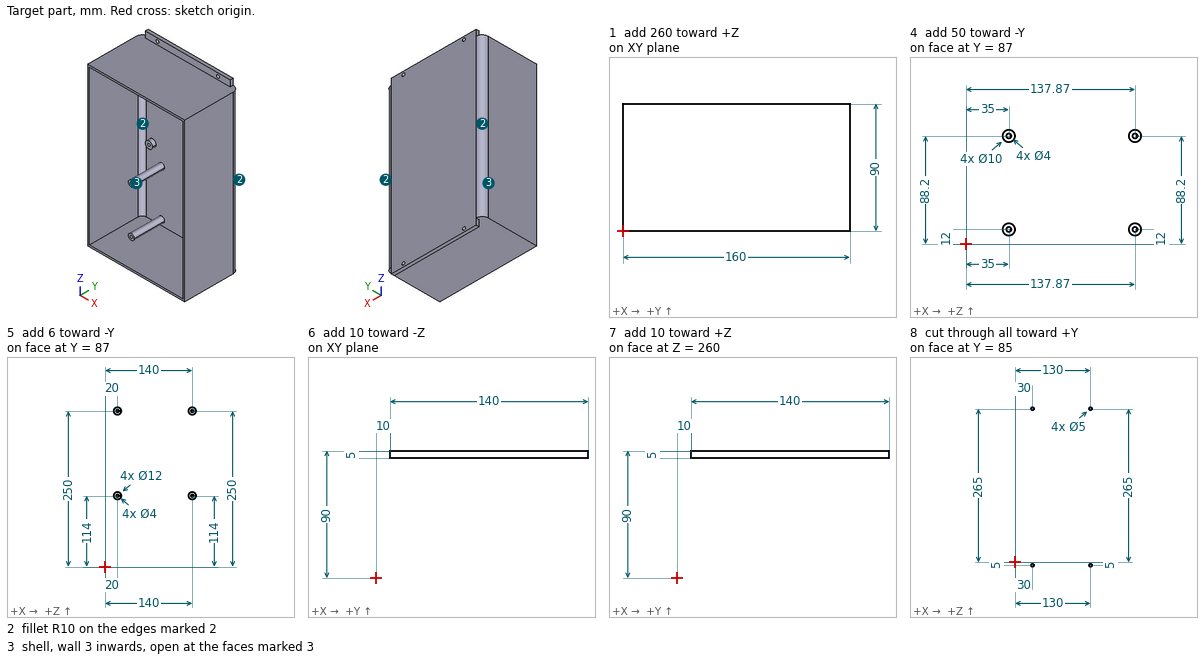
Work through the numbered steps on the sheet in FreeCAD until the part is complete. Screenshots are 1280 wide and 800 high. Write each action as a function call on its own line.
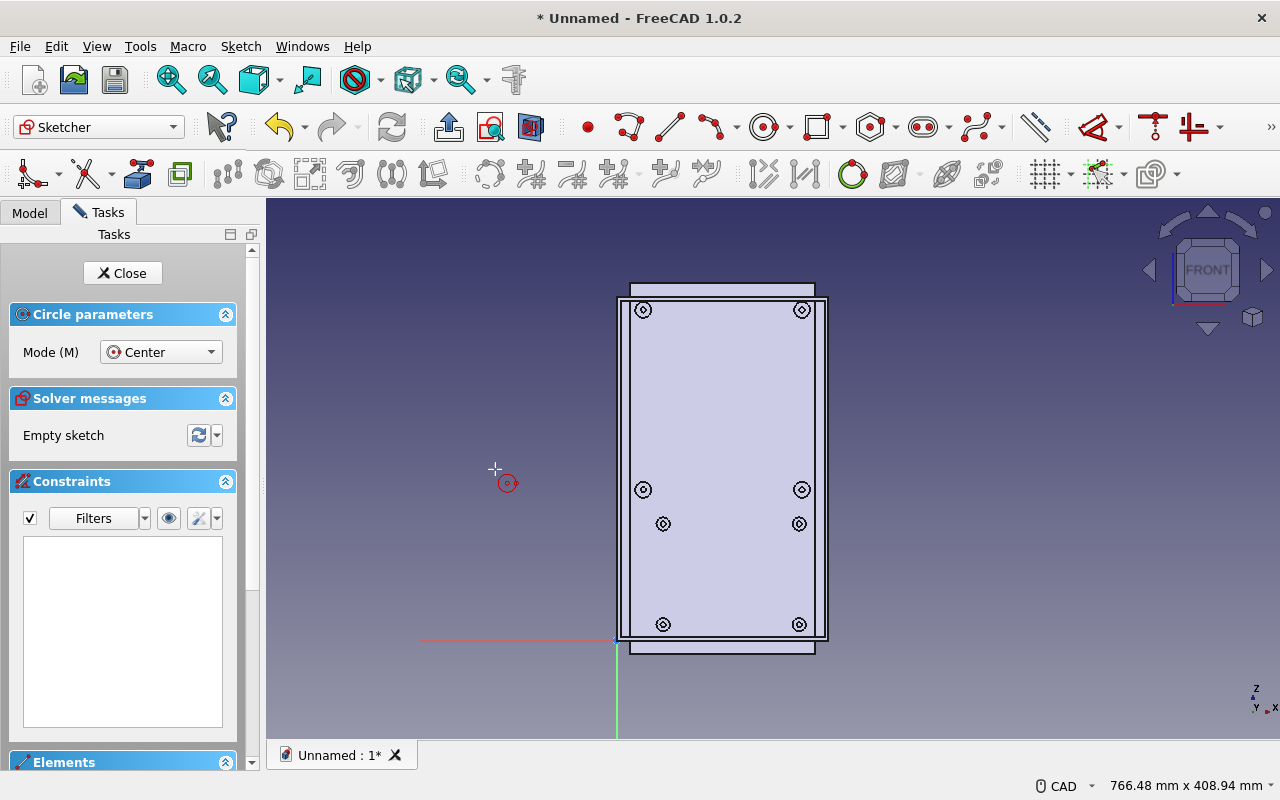
scroll(789, 290, up, 10)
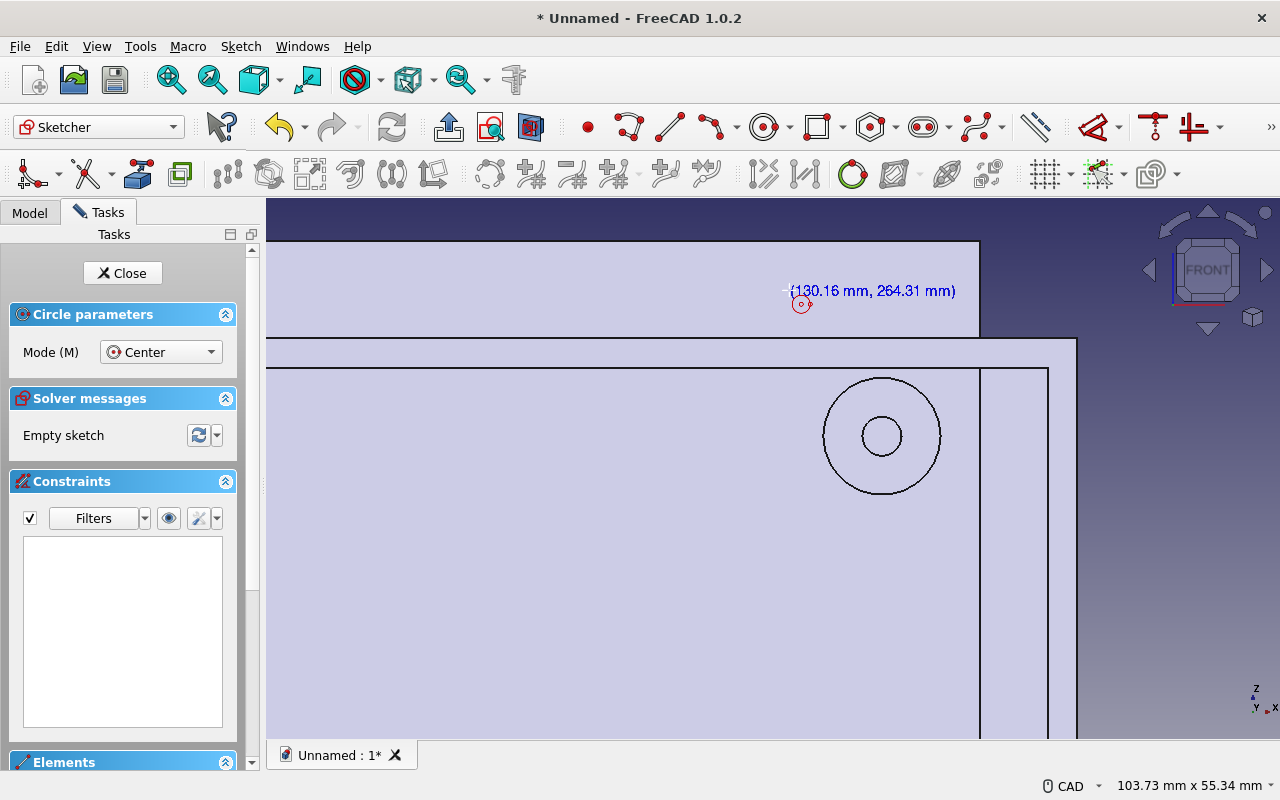
scroll(790, 290, down, 10)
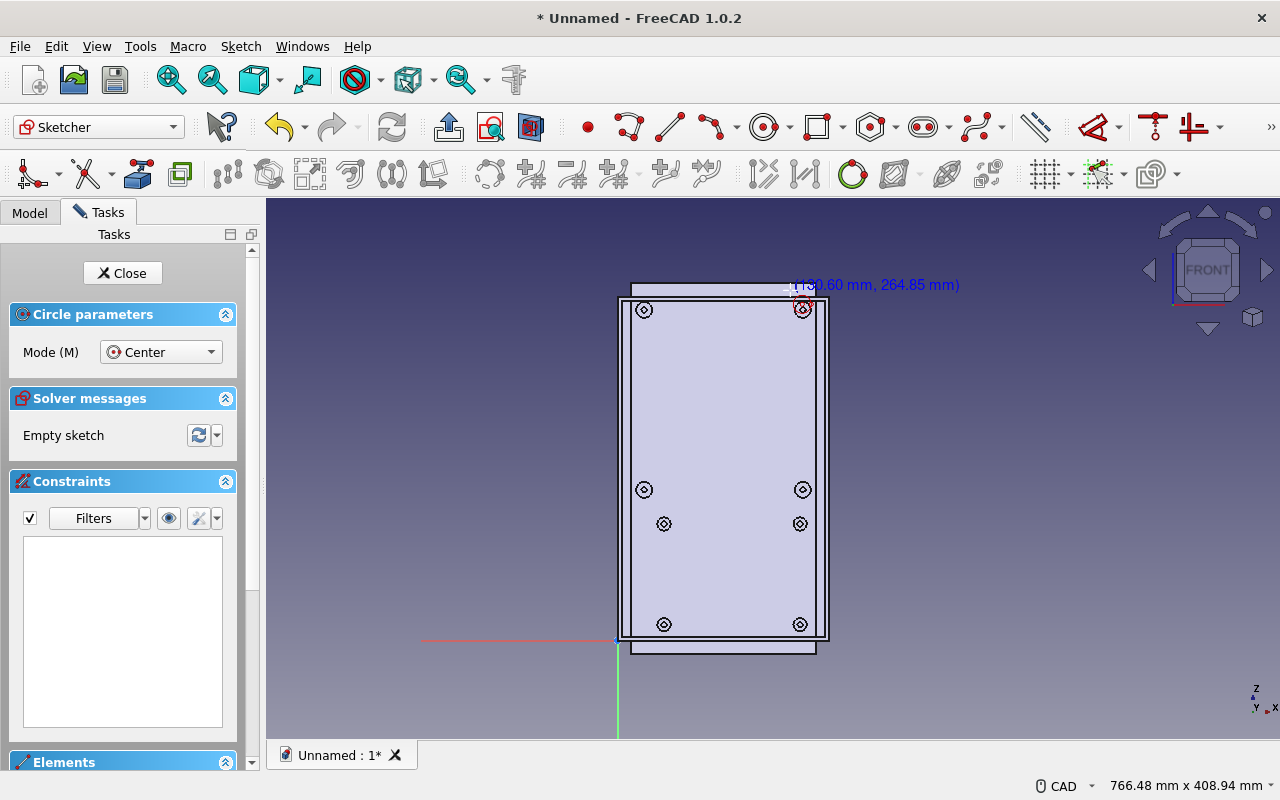
click(790, 290)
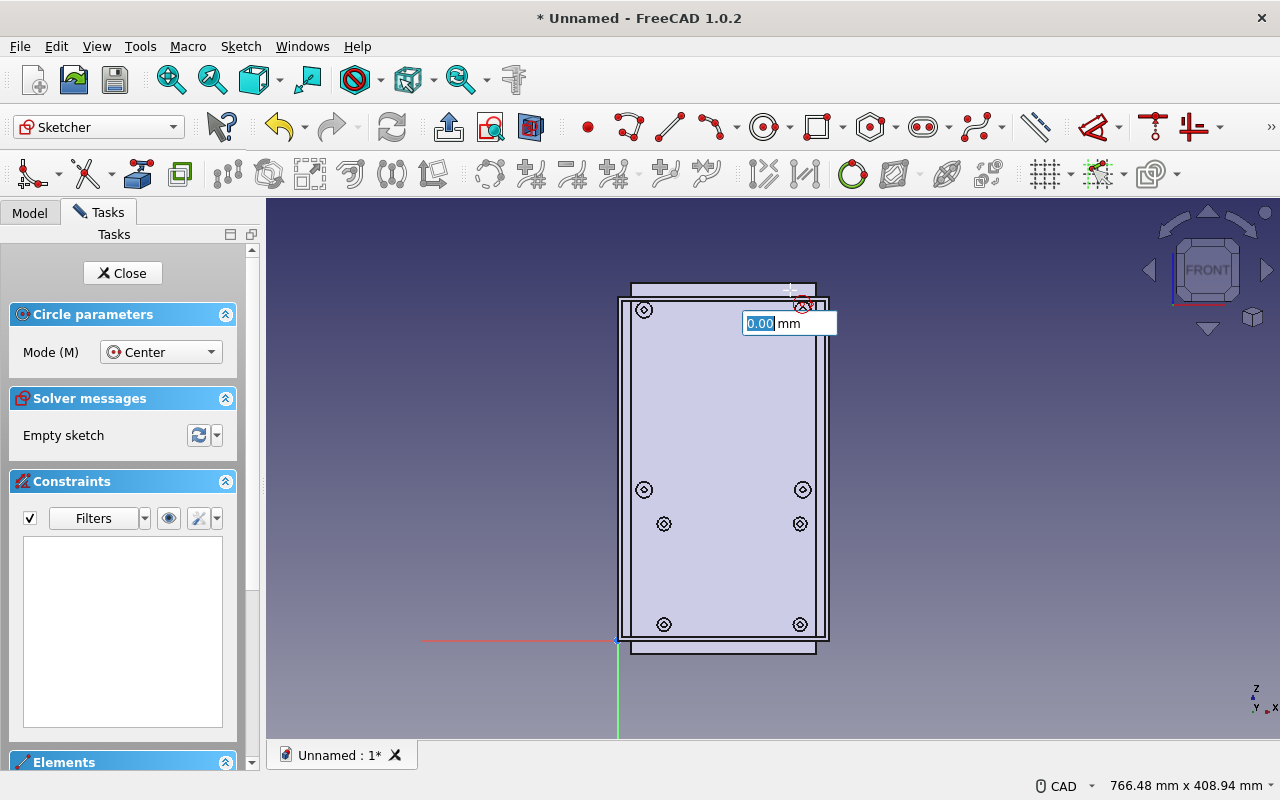
scroll(792, 288, up, 8)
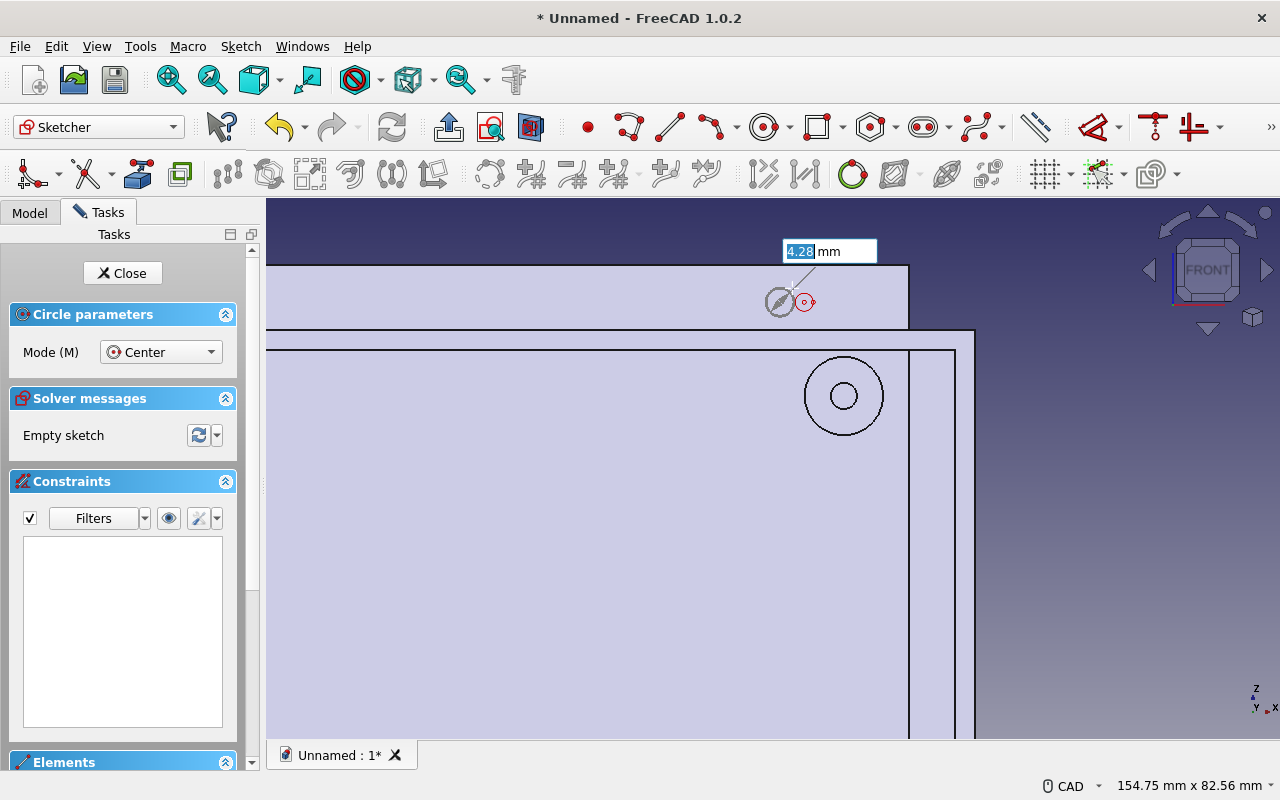
click(790, 286)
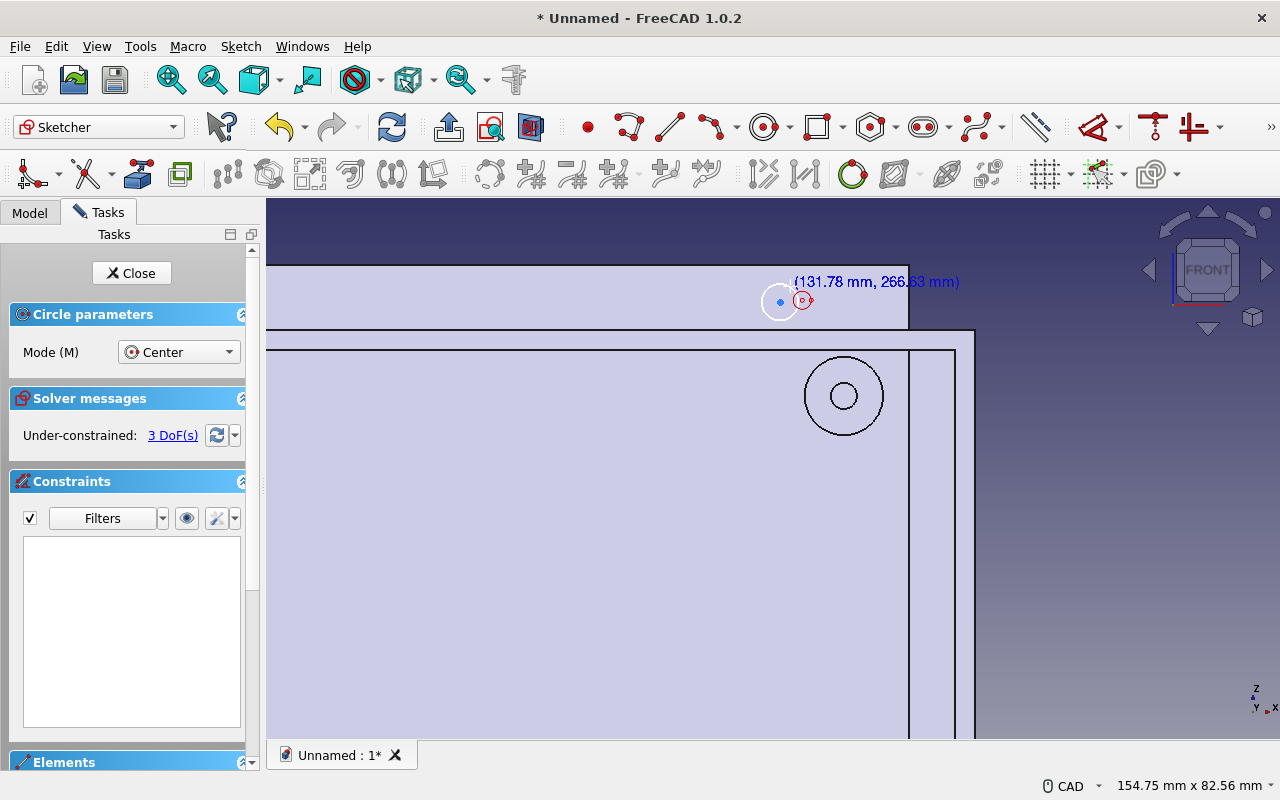
scroll(791, 288, down, 8)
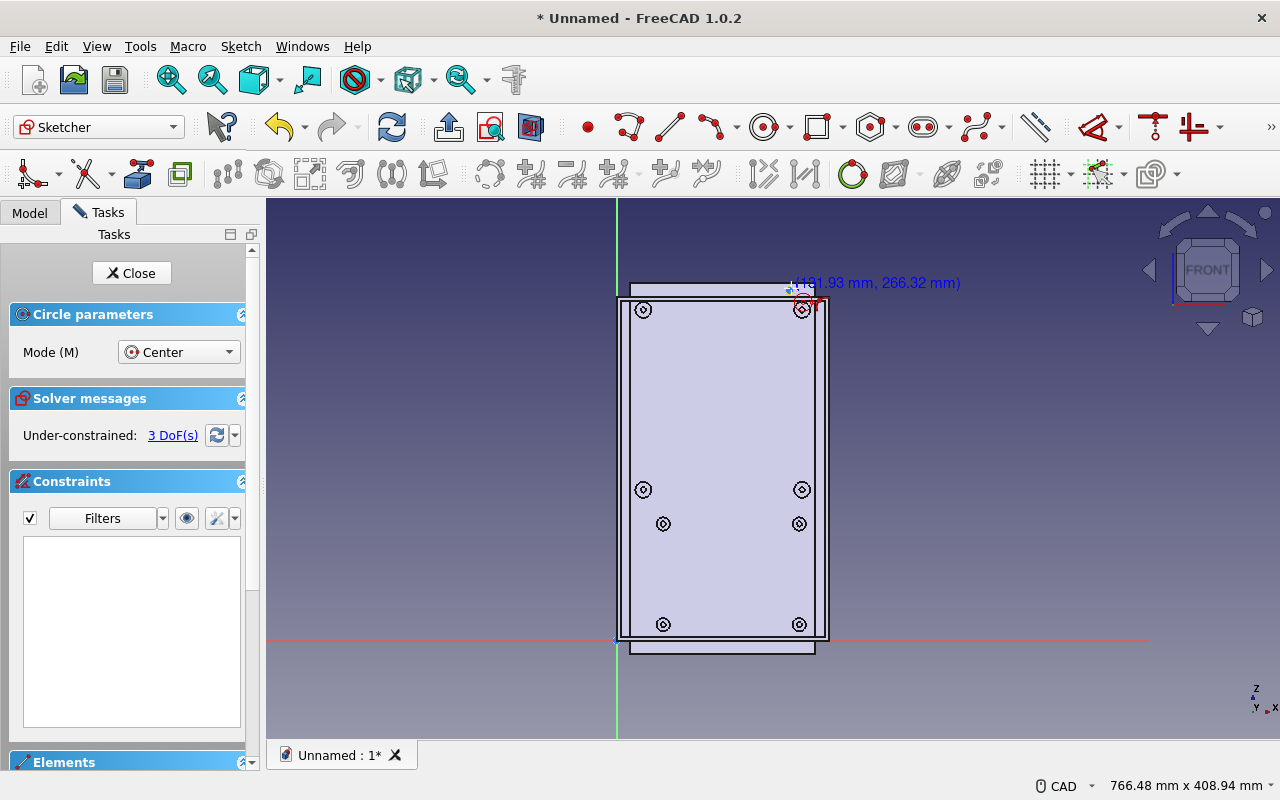
scroll(657, 290, up, 10)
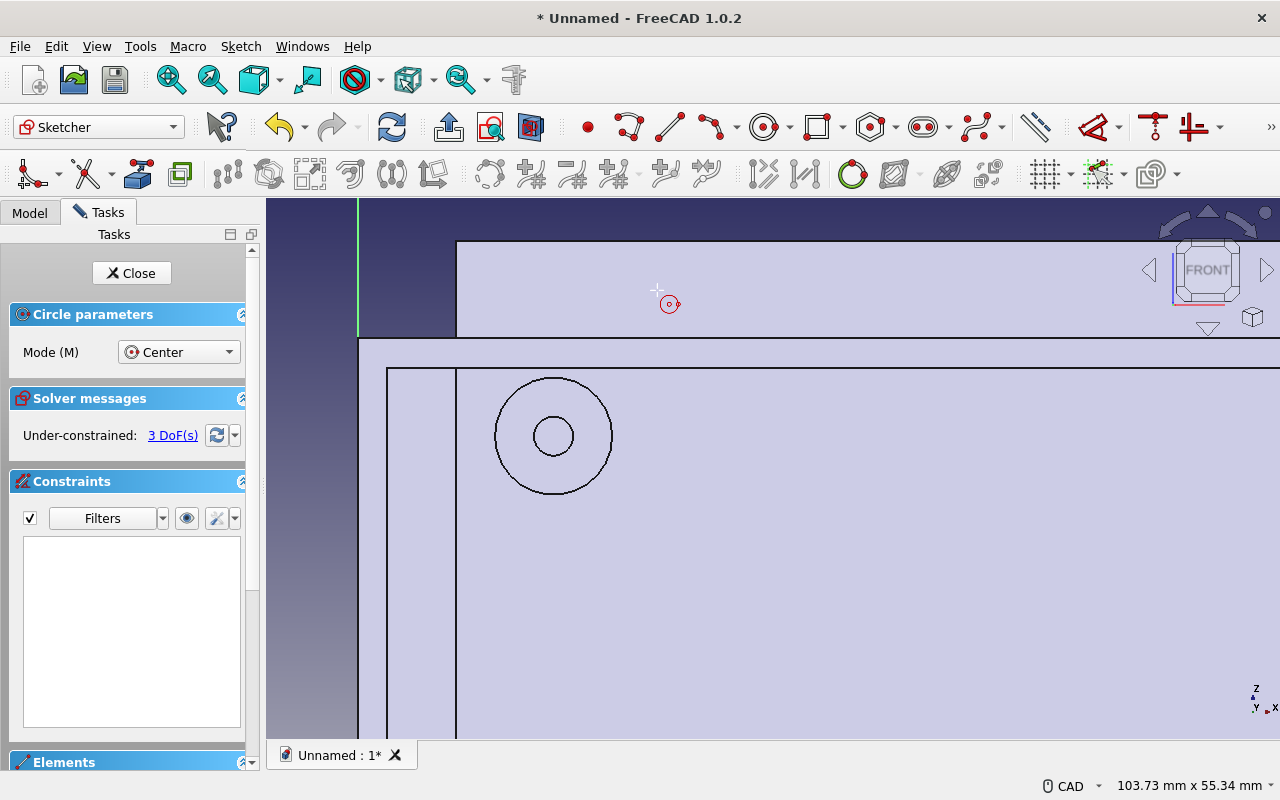
scroll(657, 290, down, 10)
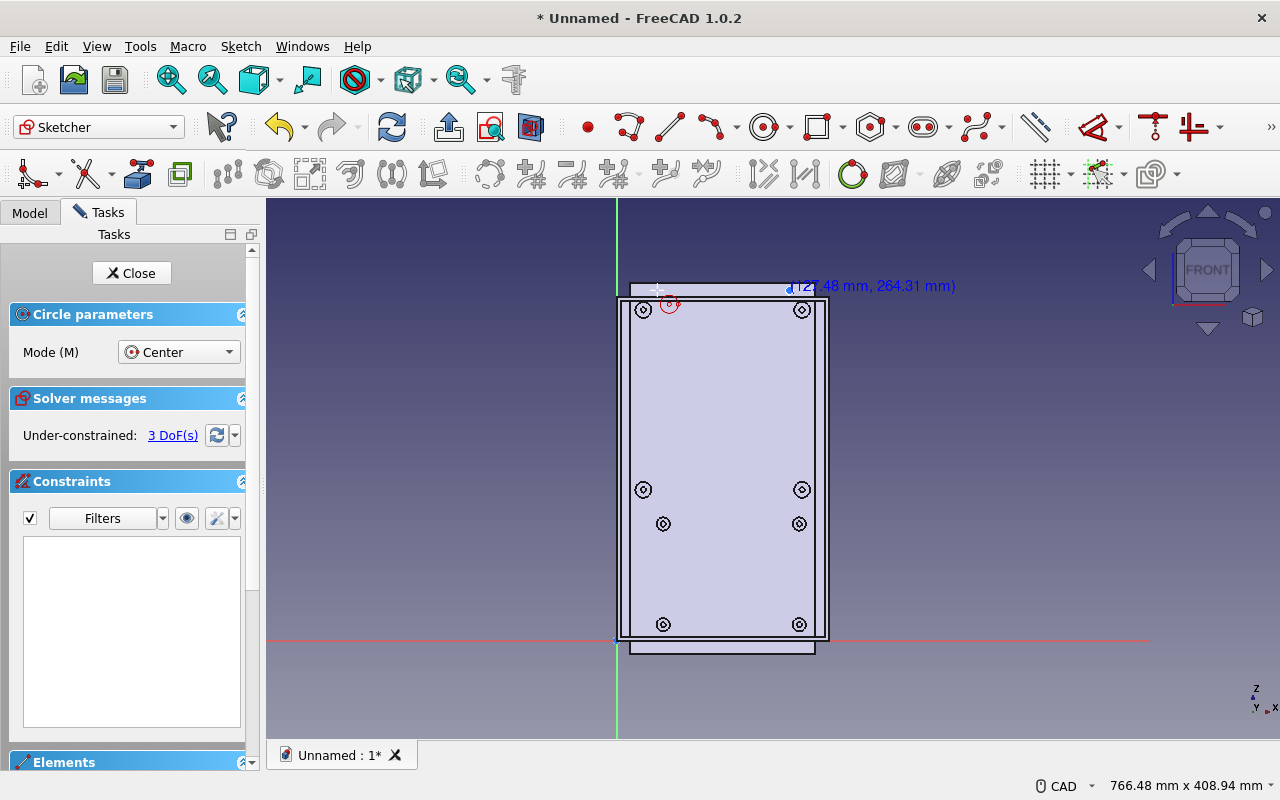
click(657, 290)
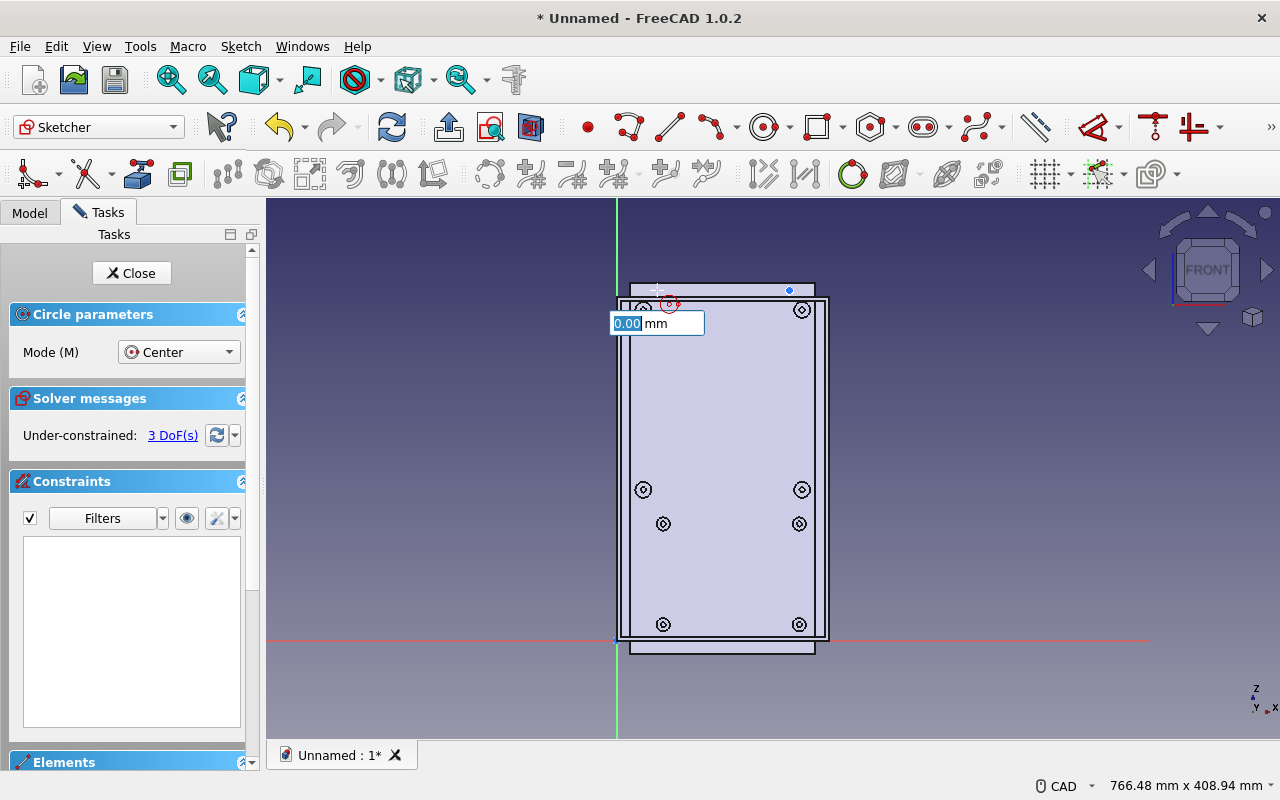
scroll(659, 288, up, 8)